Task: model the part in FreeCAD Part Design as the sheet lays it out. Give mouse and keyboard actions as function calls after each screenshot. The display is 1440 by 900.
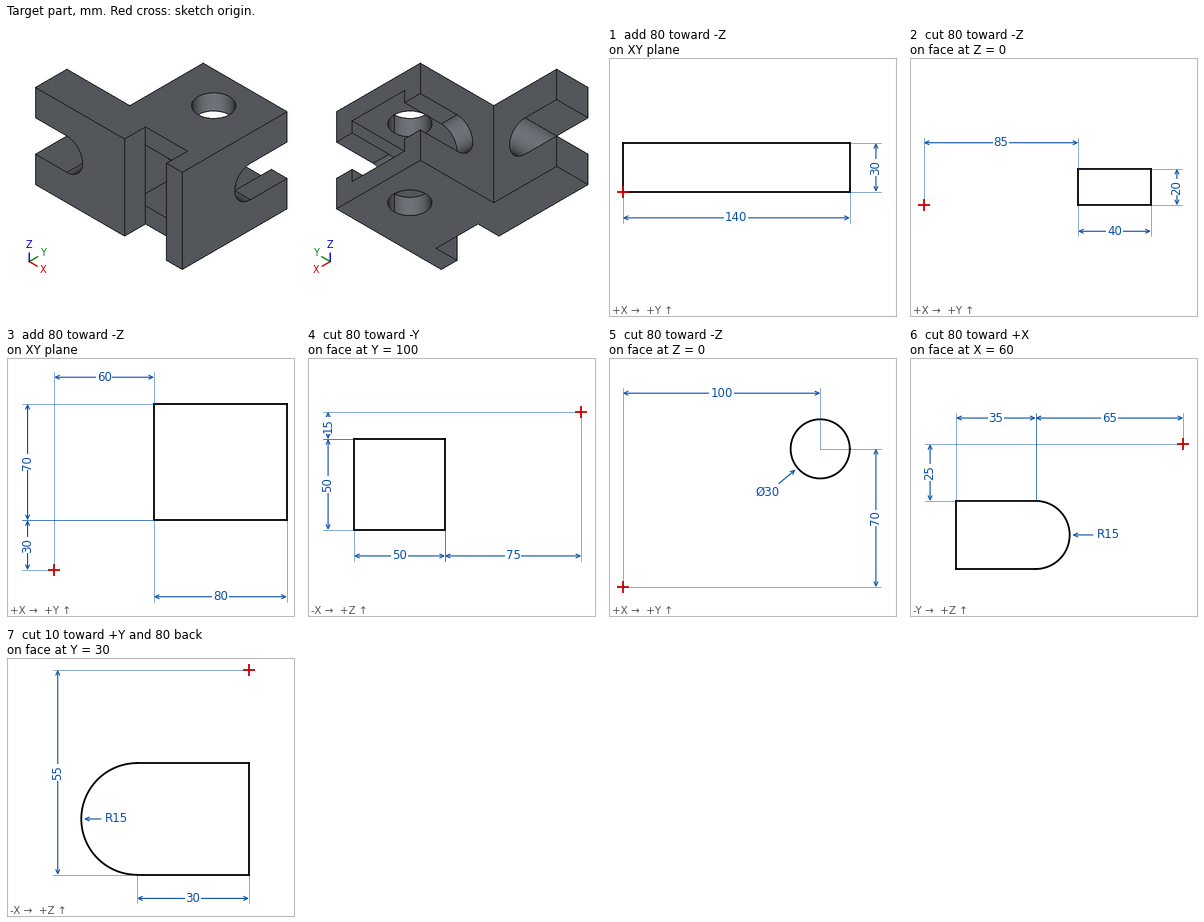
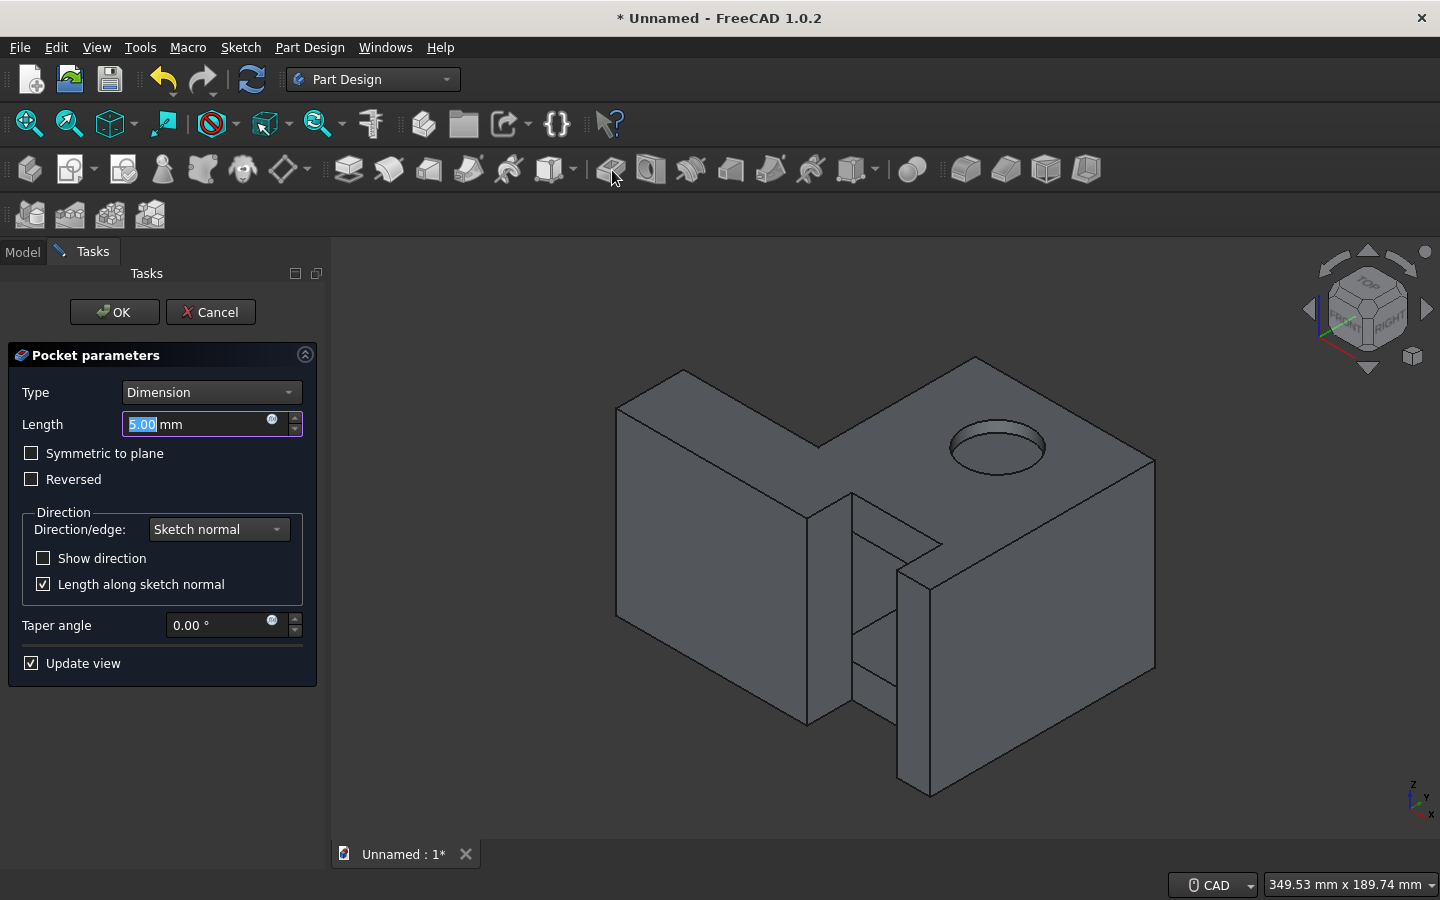
text(80)
key(Tab)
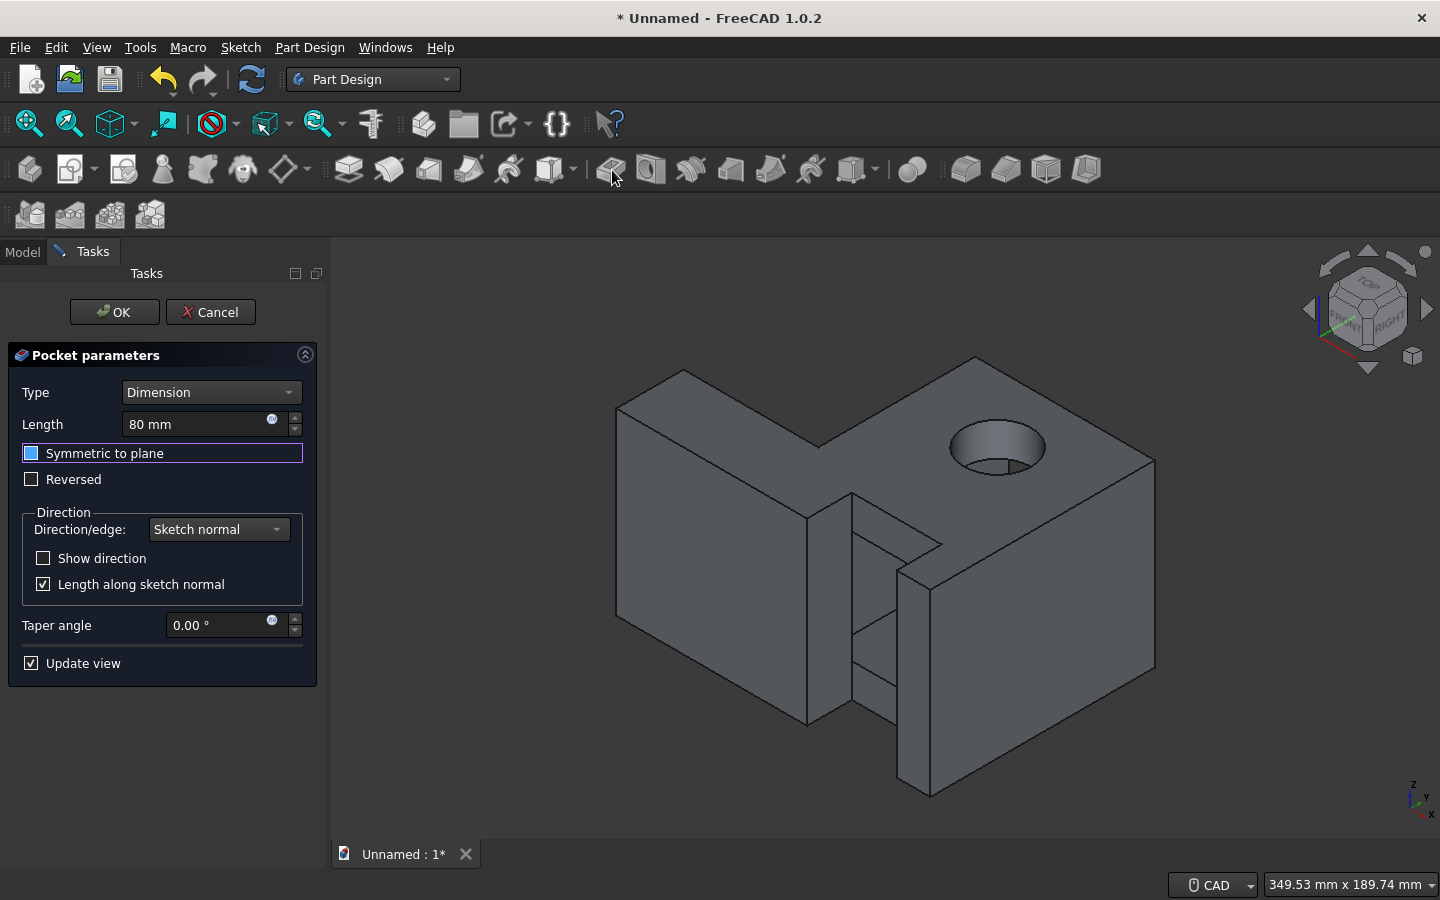
click(115, 312)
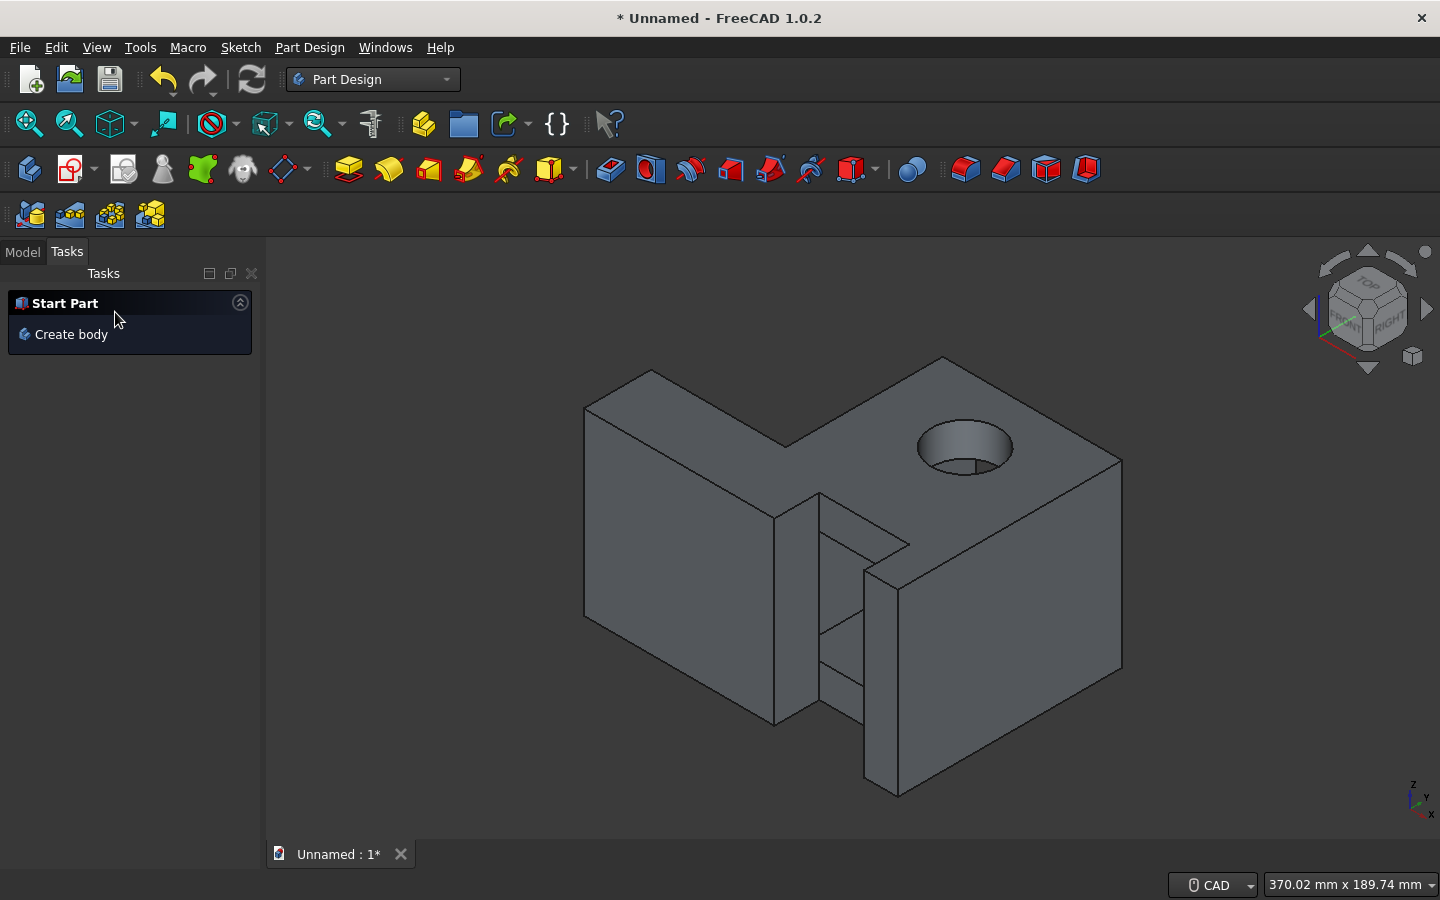
key(6)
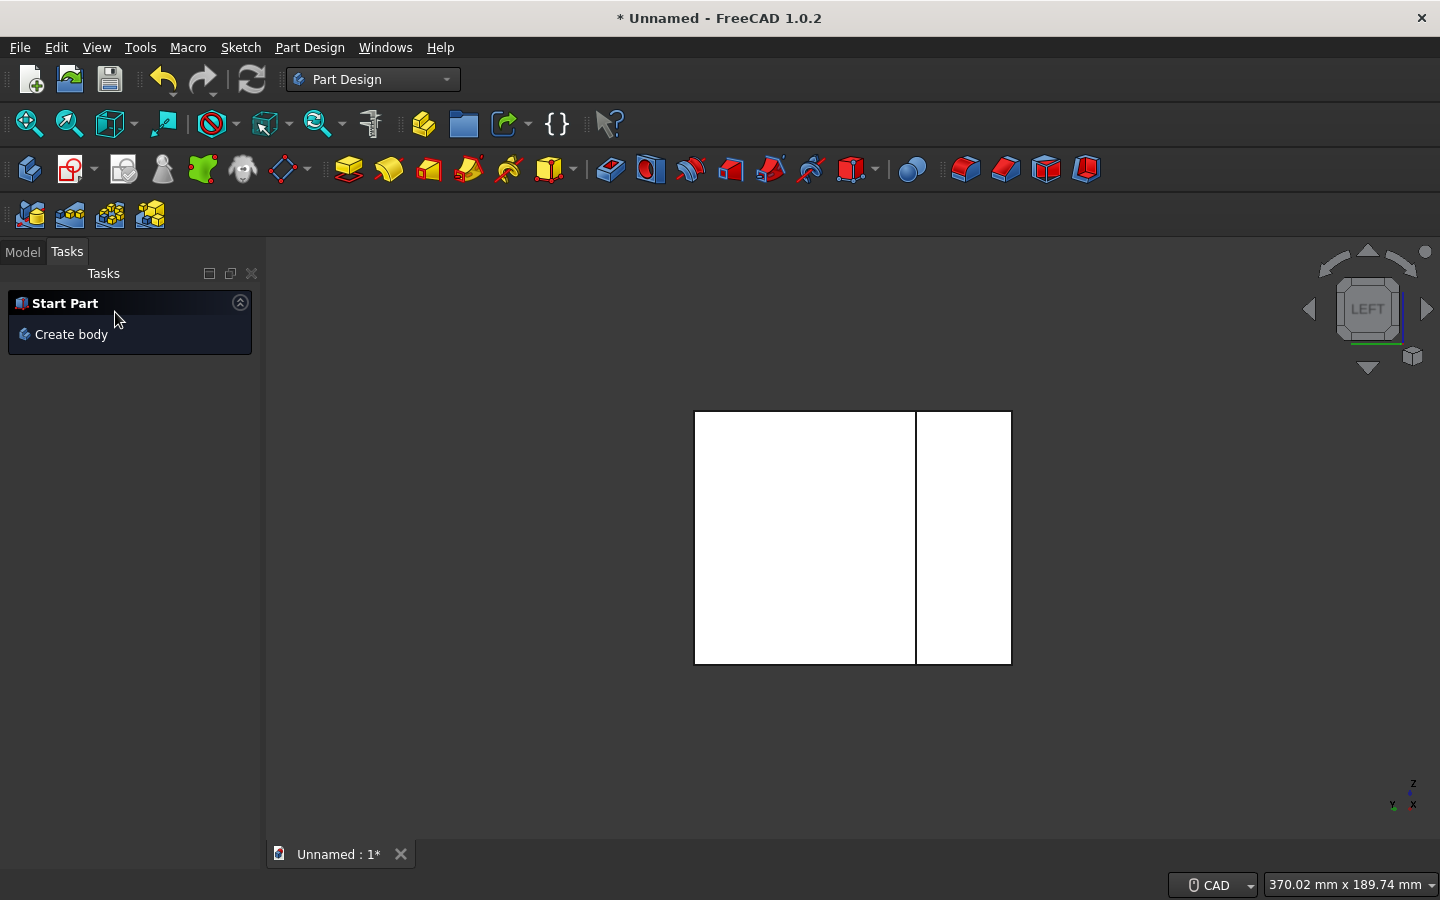
key(v)
key(f)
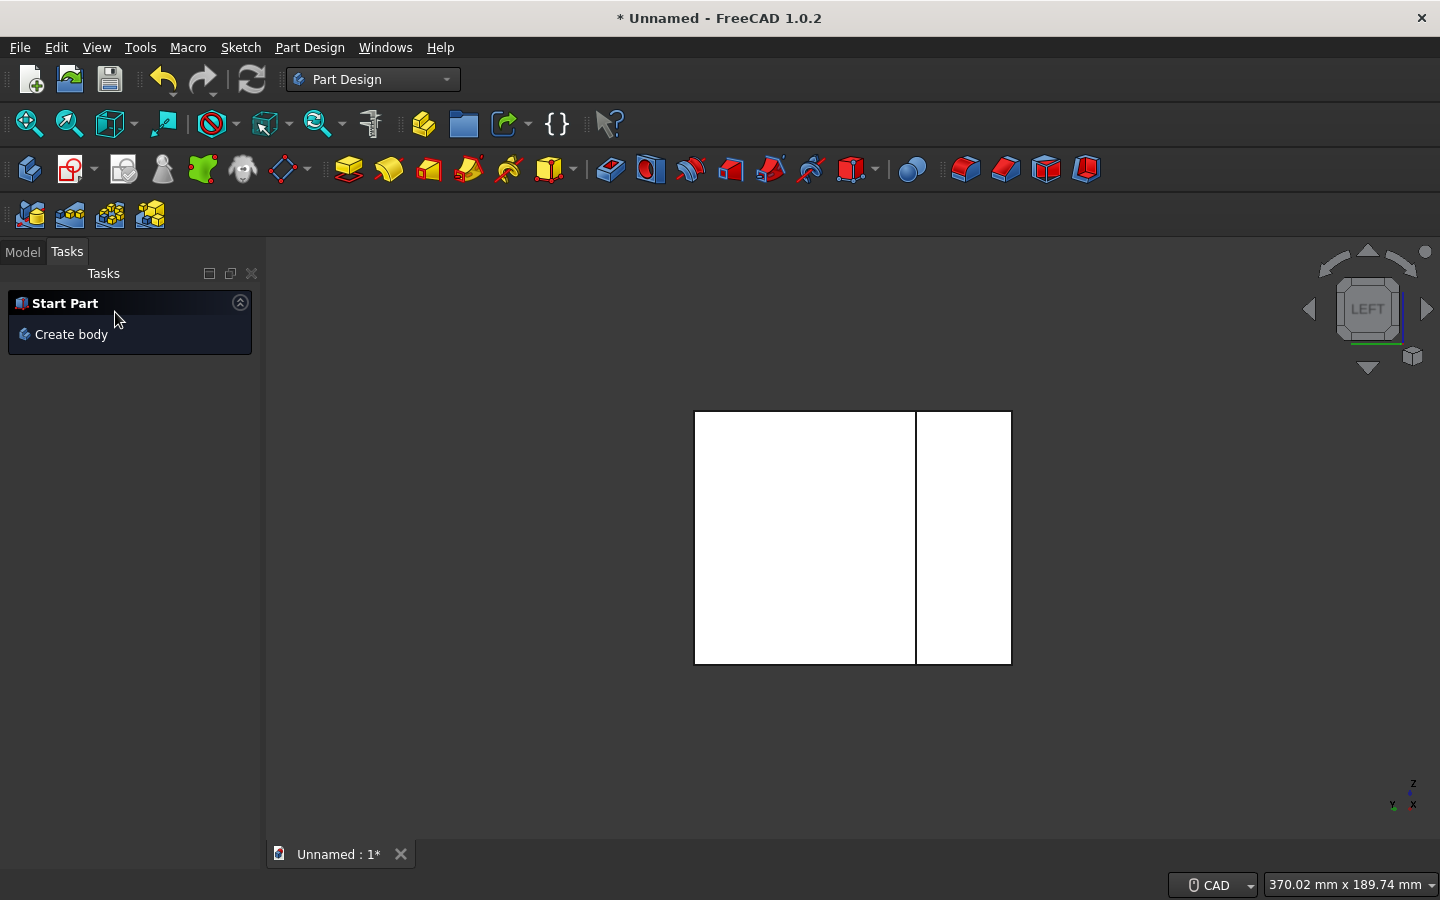
click(805, 537)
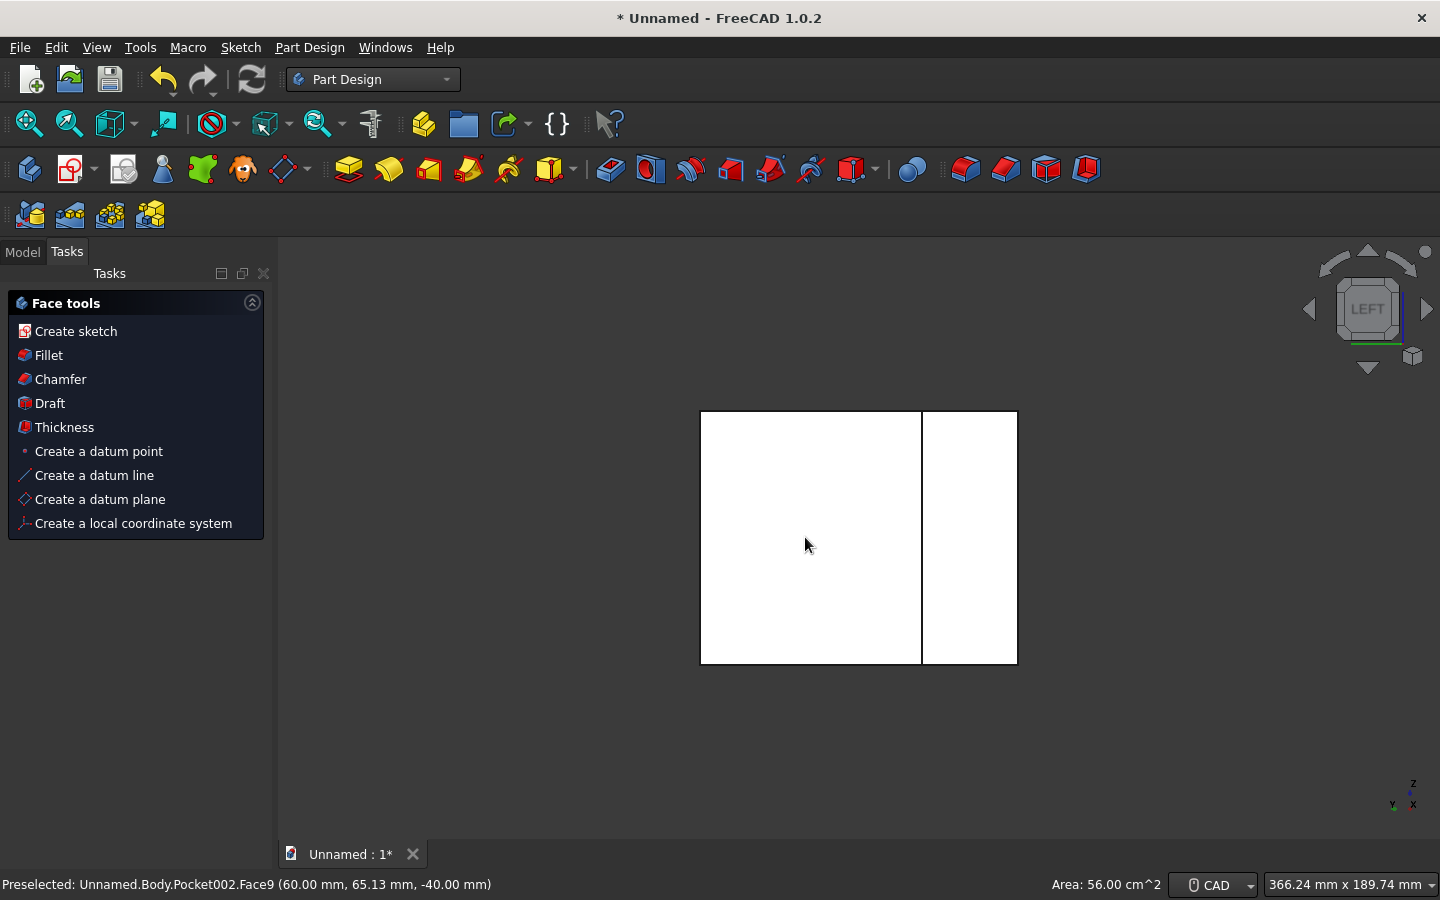
click(70, 170)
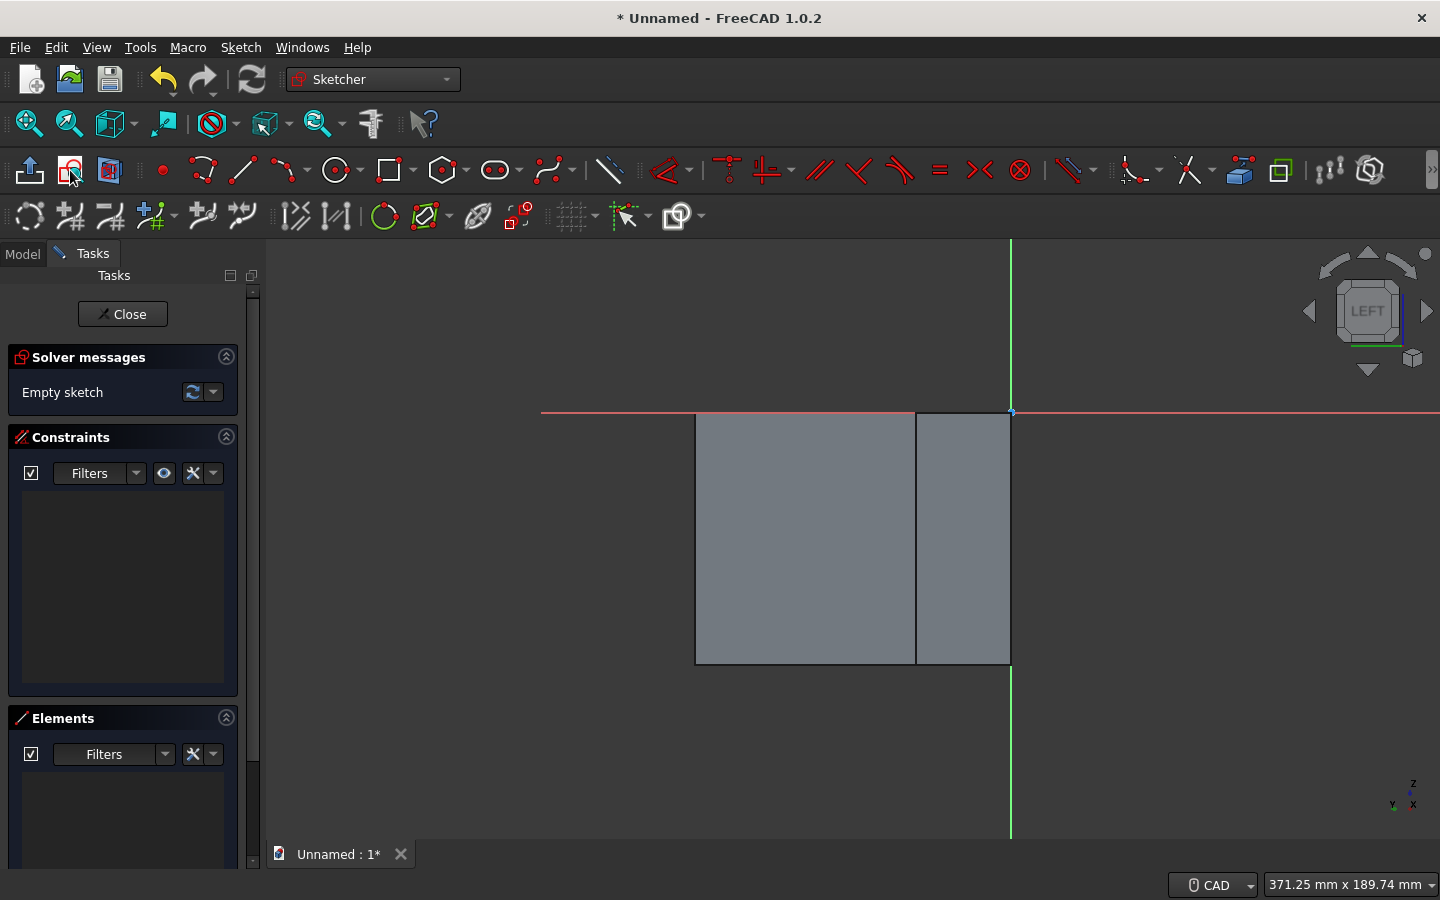
scroll(909, 467, up, 4)